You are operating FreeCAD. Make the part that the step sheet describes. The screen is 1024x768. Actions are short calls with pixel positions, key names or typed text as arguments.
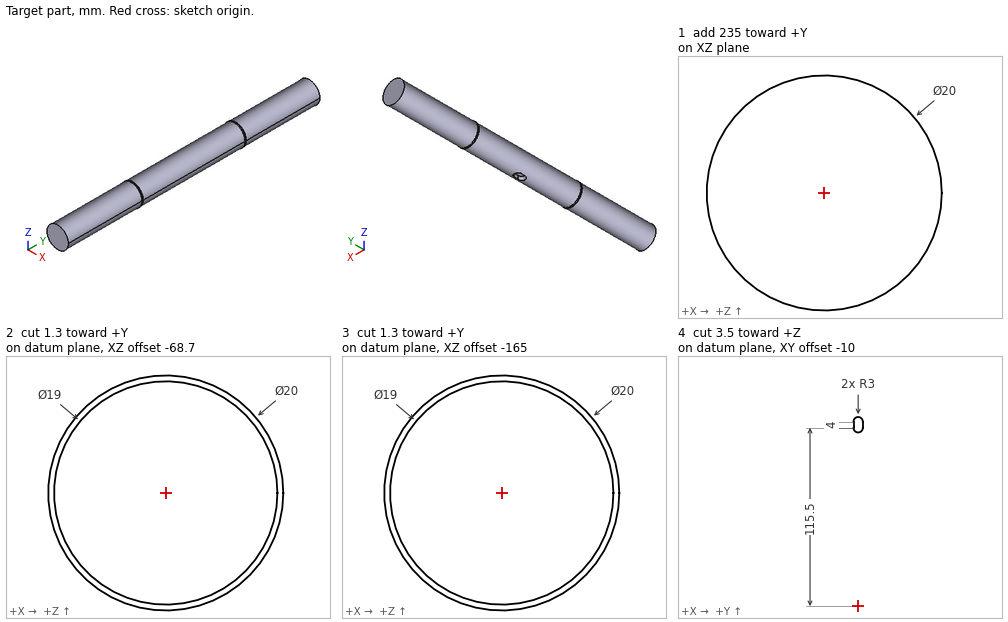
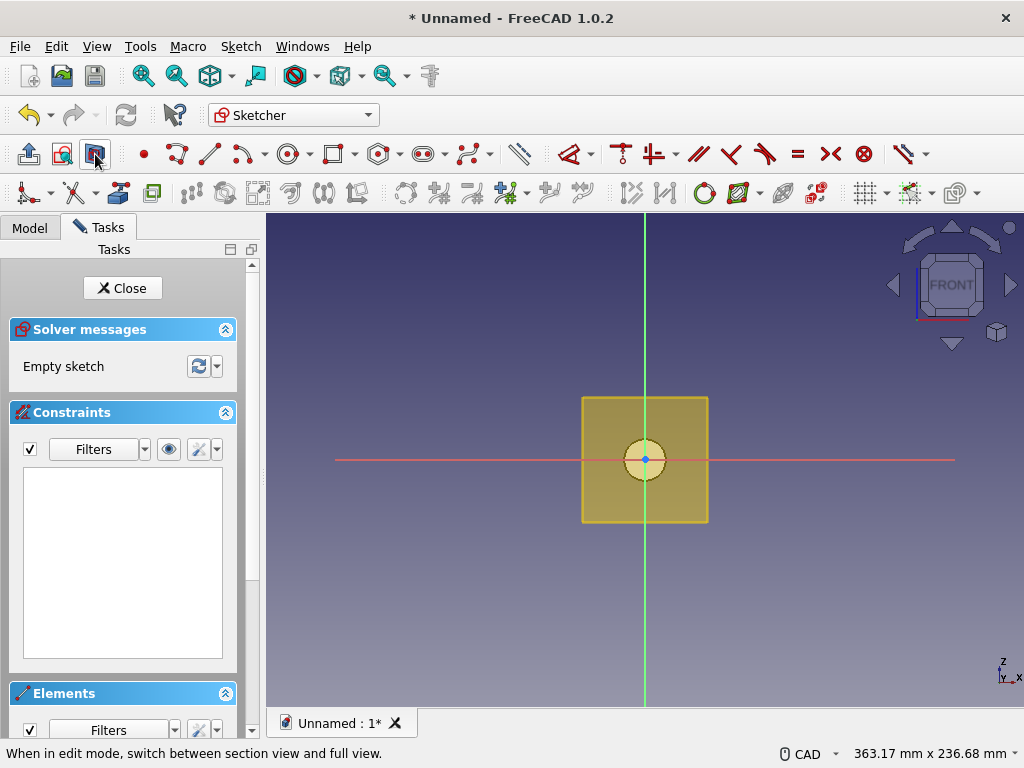
scroll(656, 460, up, 10)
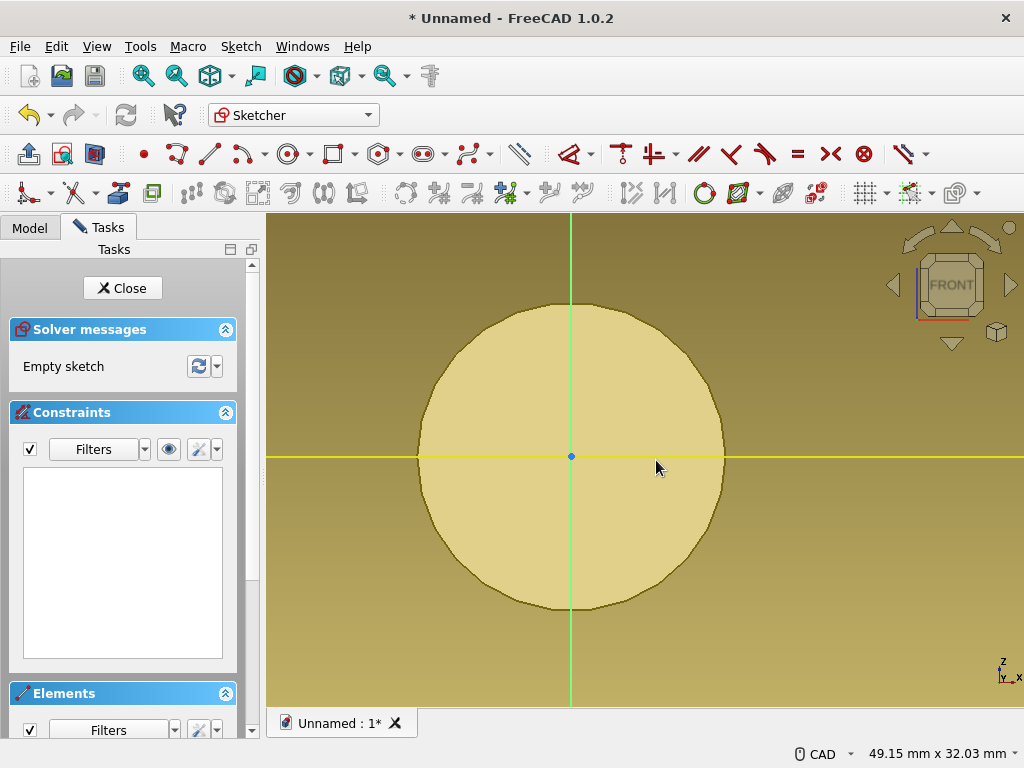
click(288, 154)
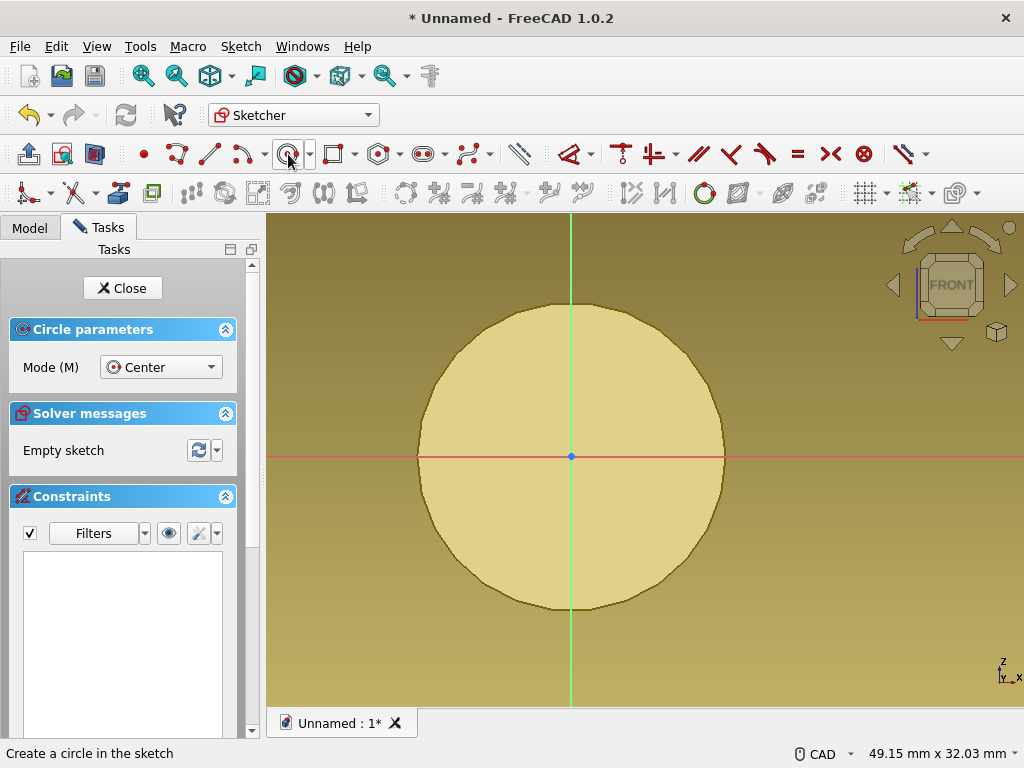
click(571, 457)
move(680, 348)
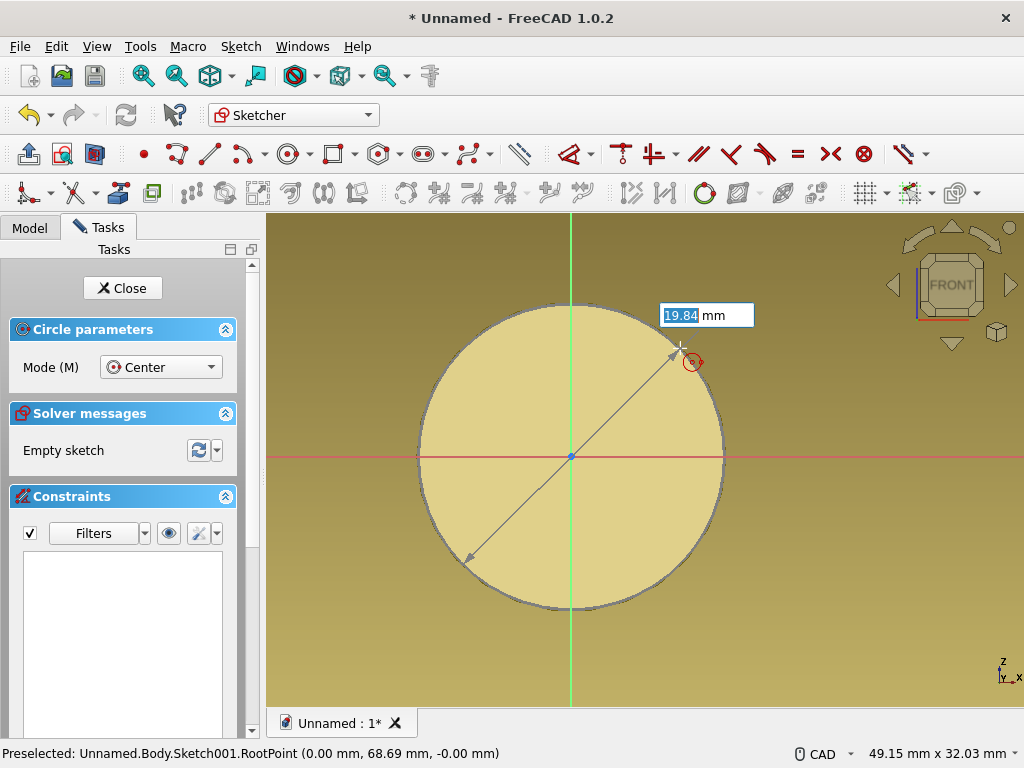
text(20)
key(Return)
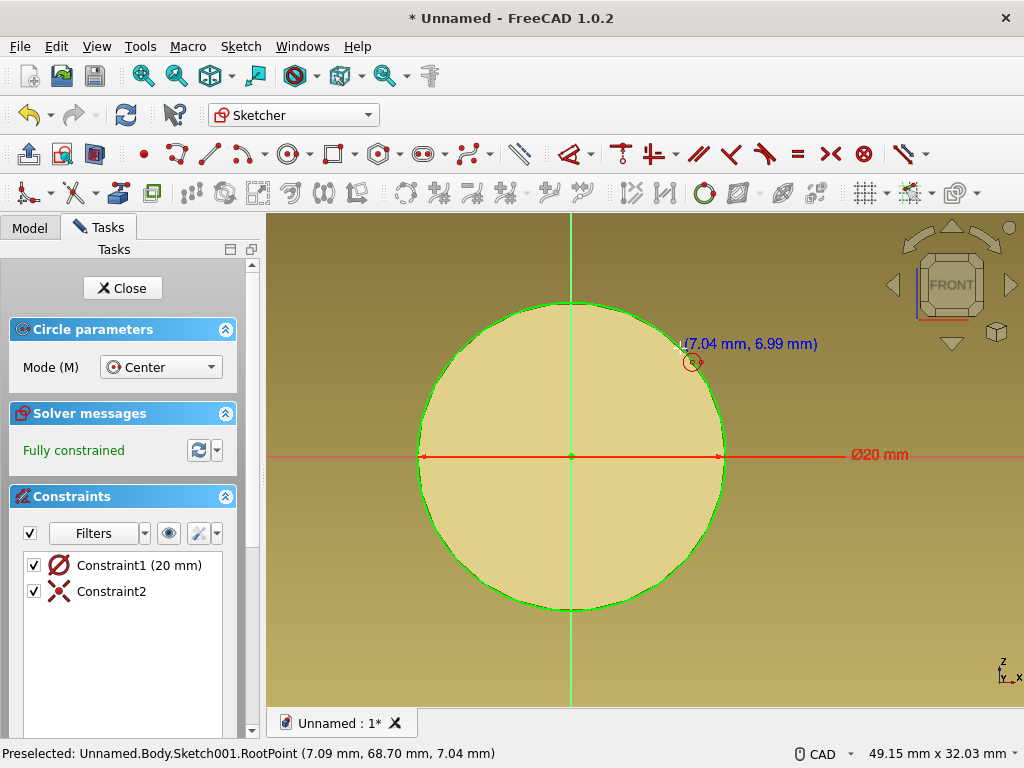
click(571, 457)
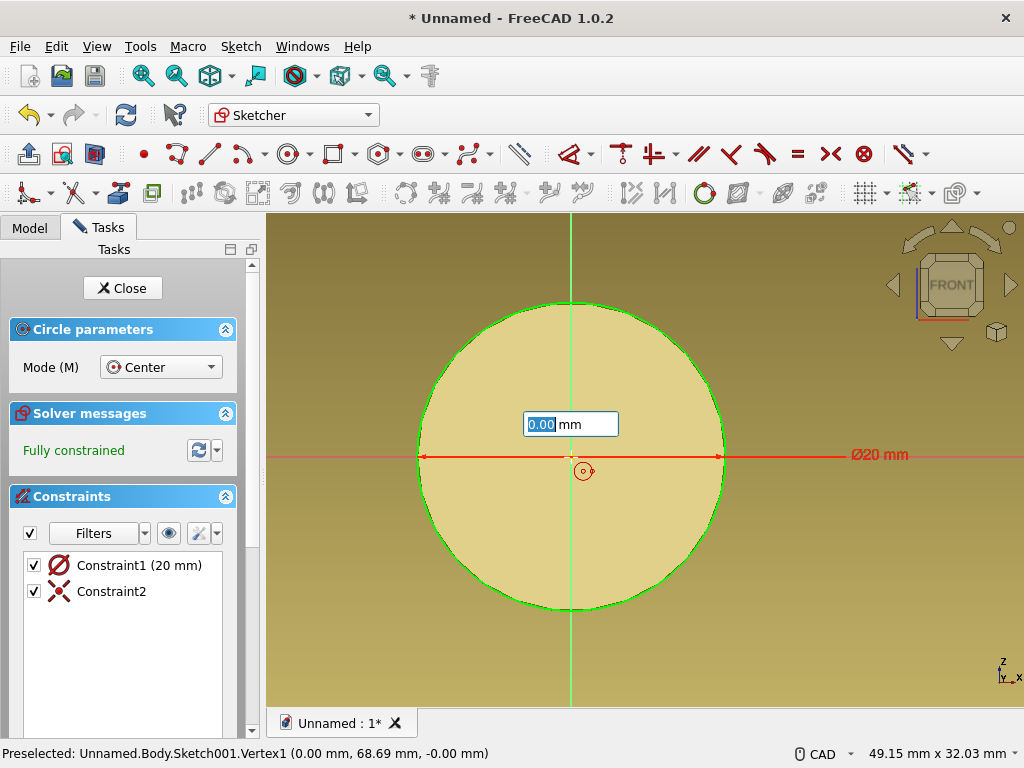
scroll(675, 353, up, 4)
move(674, 353)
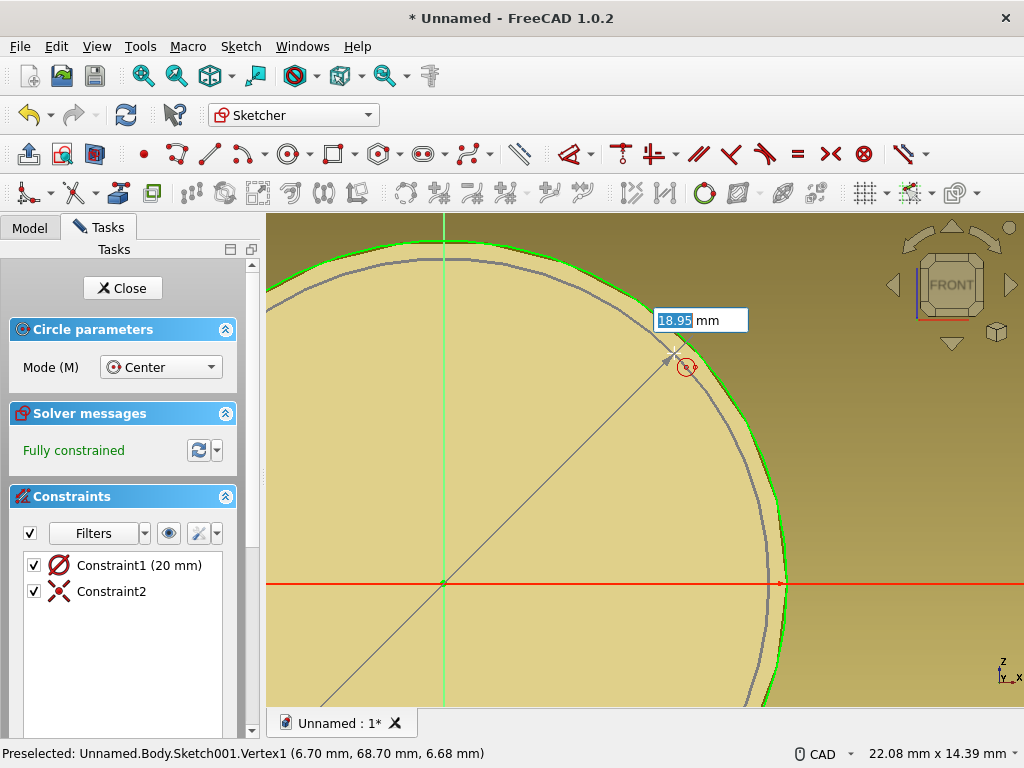
text(19)
key(Return)
key(Escape)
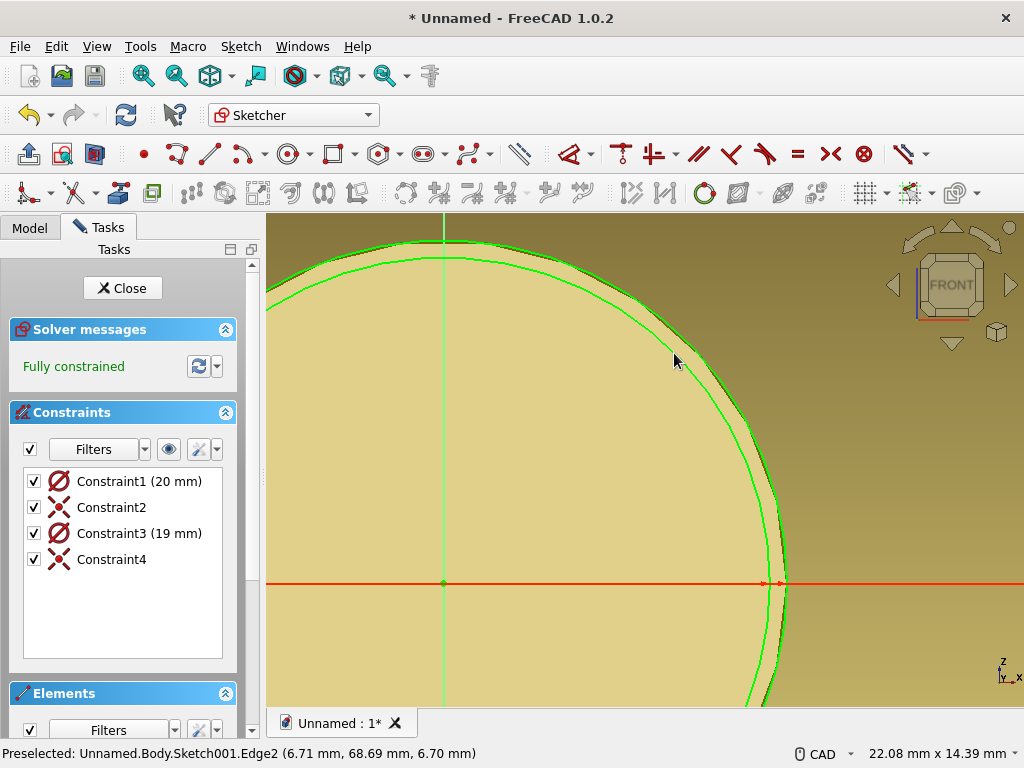
click(123, 288)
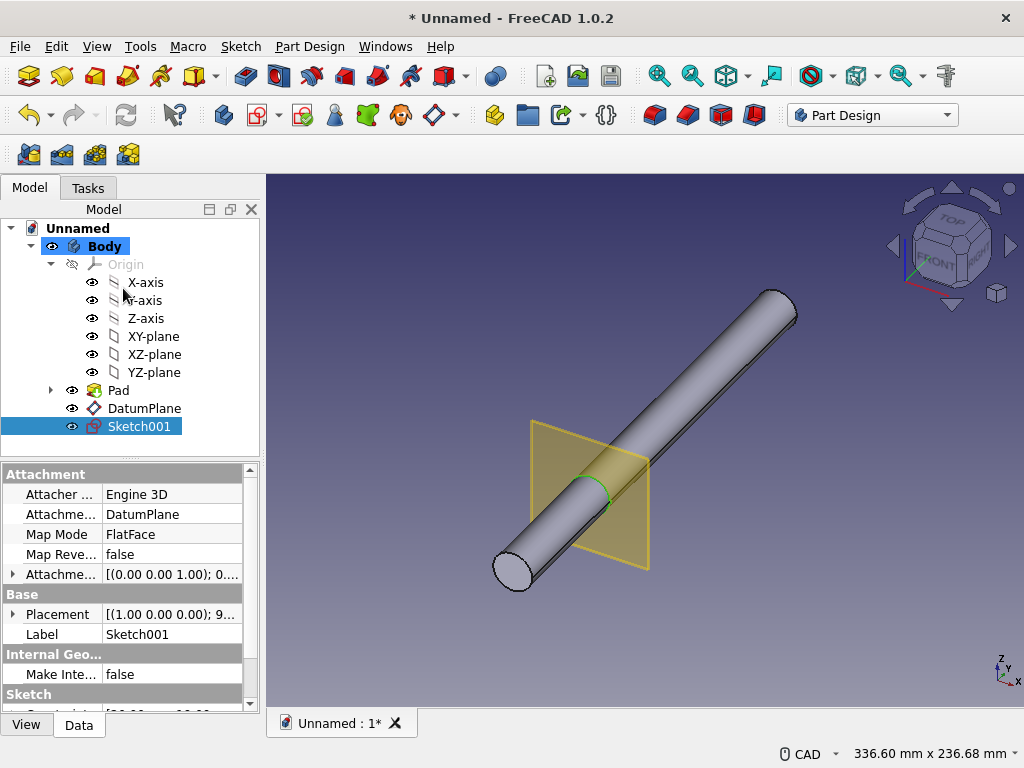
click(246, 76)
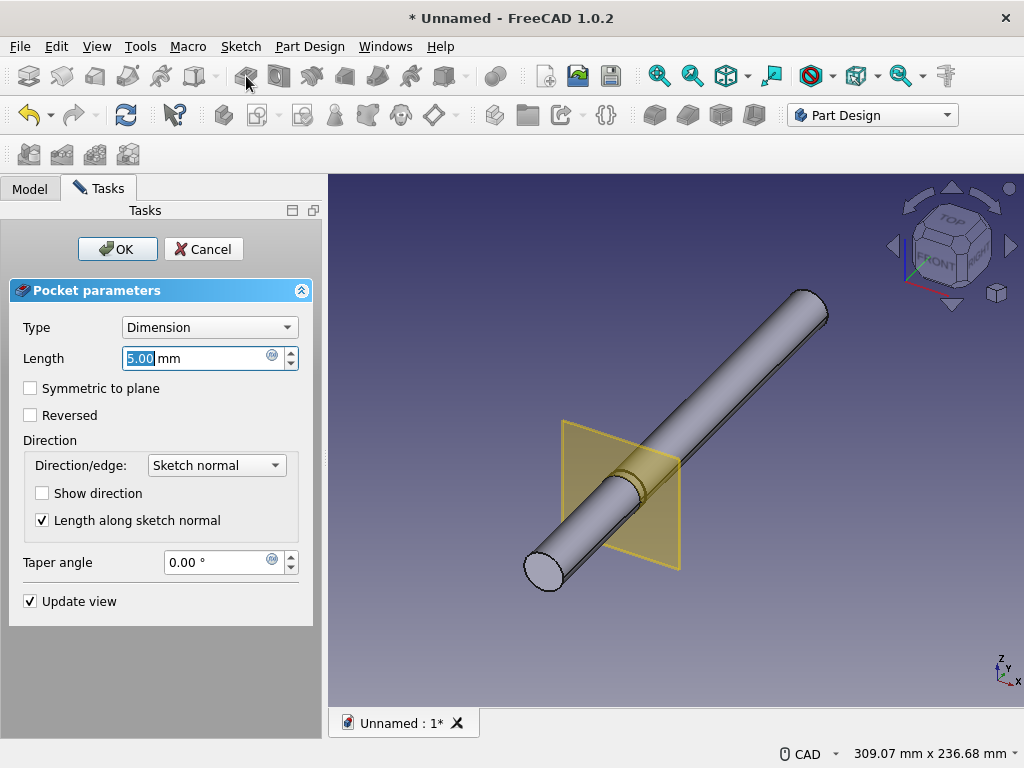
text(1.3)
key(Tab)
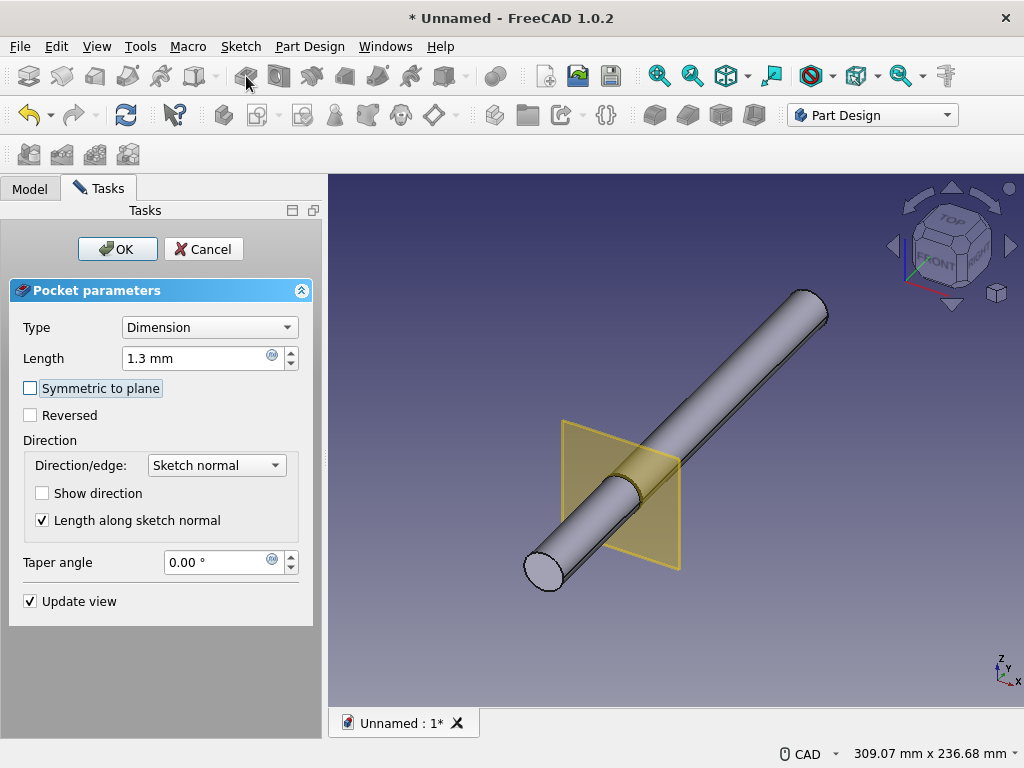
click(118, 249)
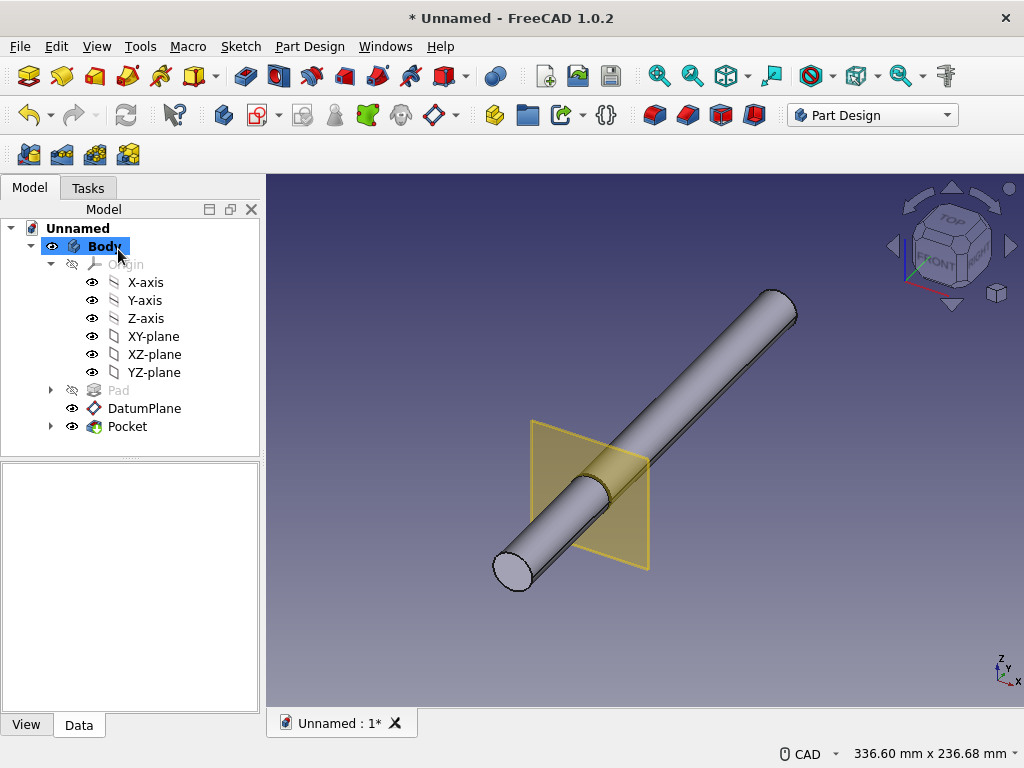
click(117, 408)
key(space)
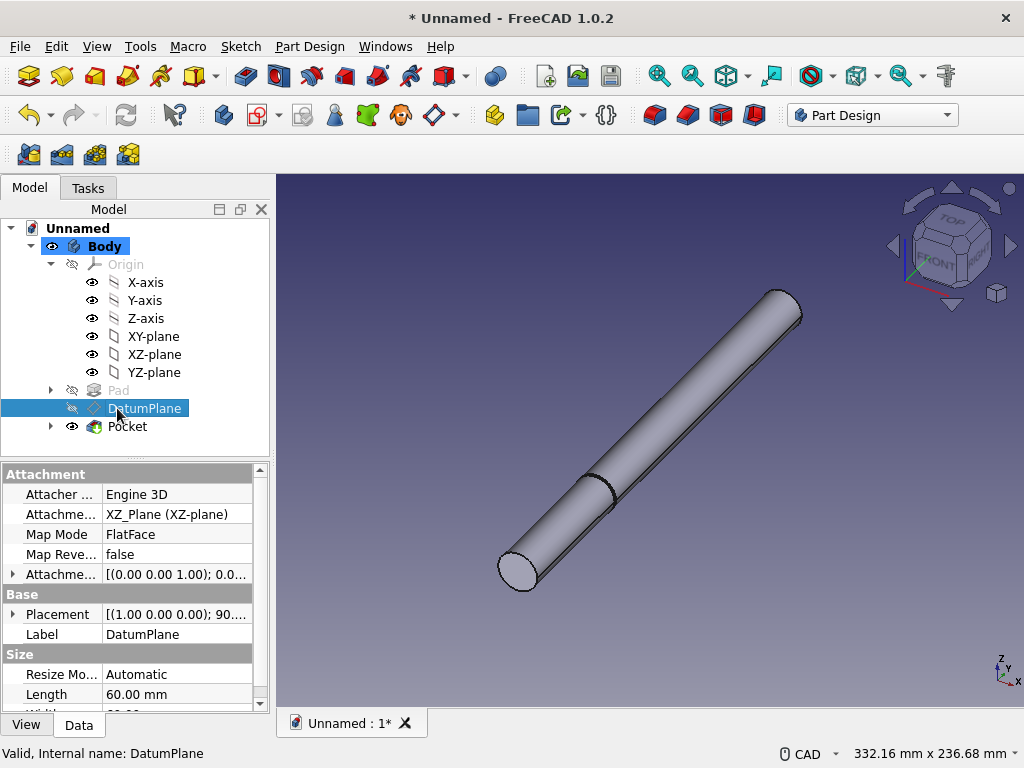
click(137, 354)